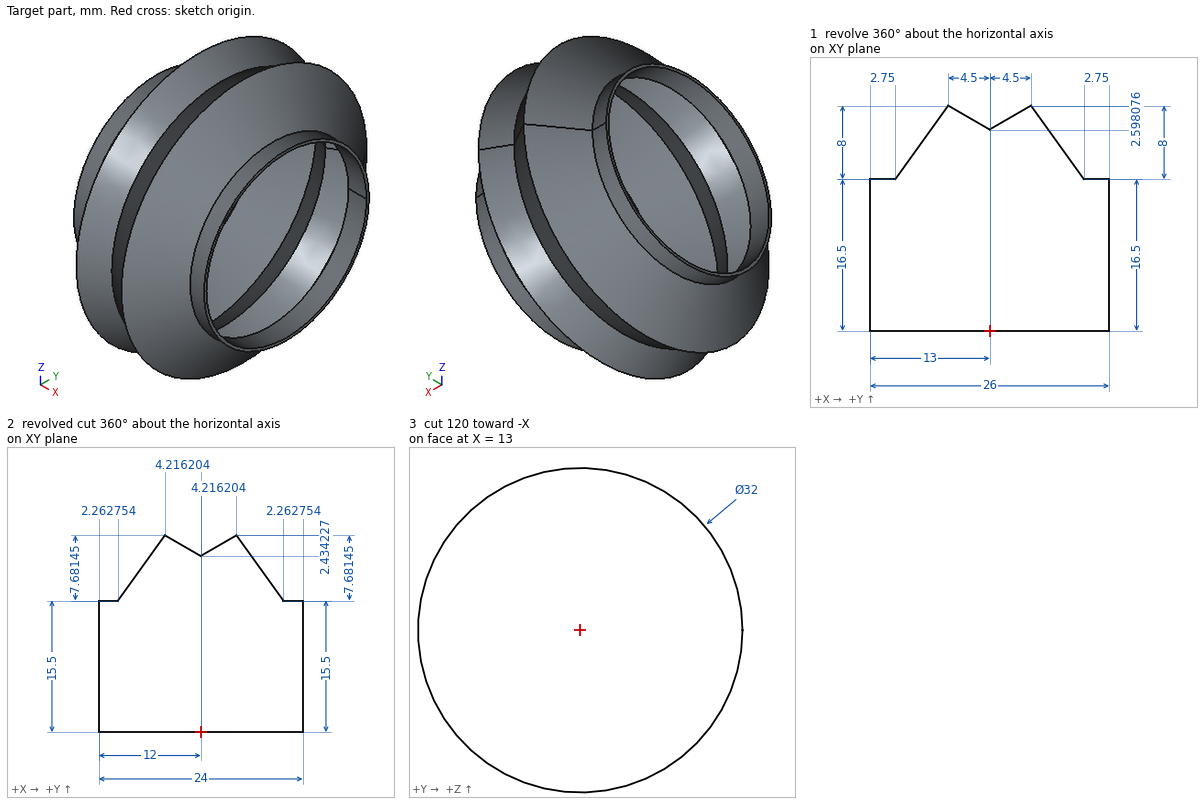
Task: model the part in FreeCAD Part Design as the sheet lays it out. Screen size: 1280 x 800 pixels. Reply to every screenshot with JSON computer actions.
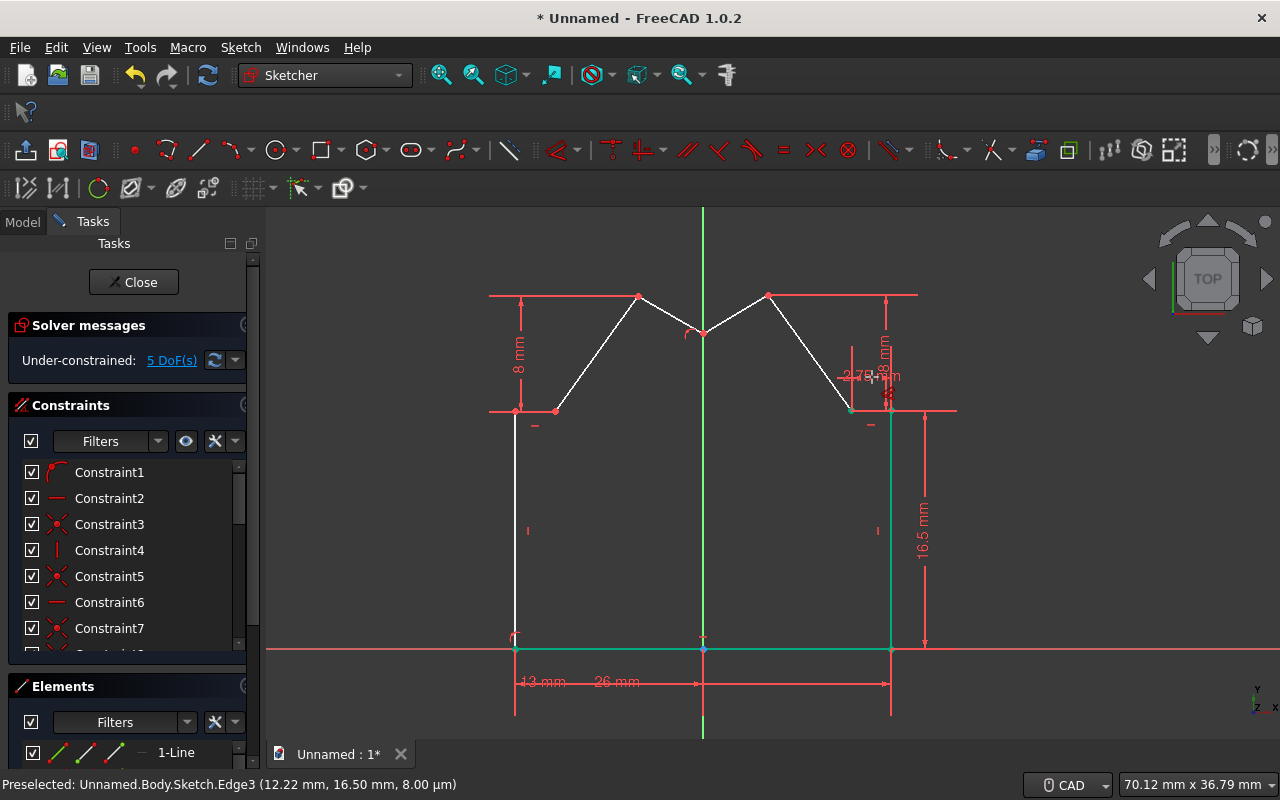
{"action": "left_click", "coordinate": [543, 412]}
{"action": "left_click", "coordinate": [535, 378]}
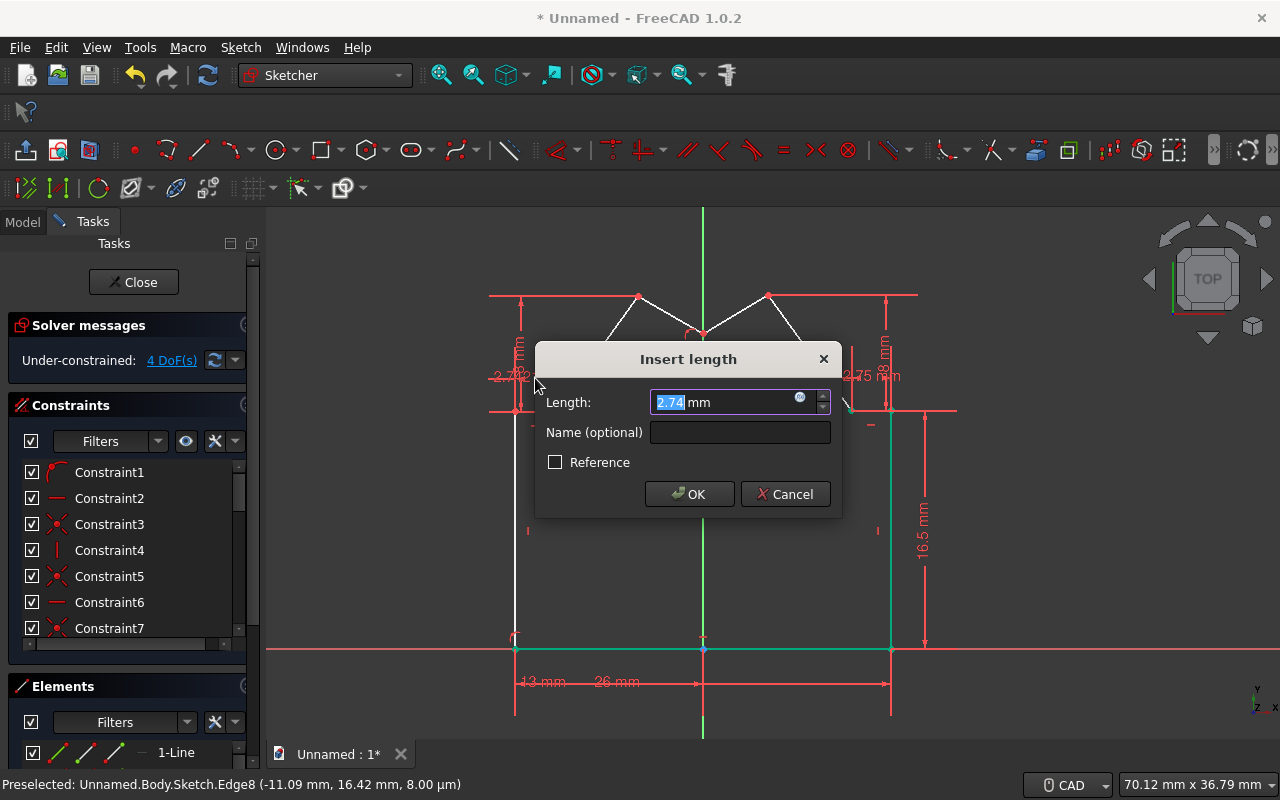
{"action": "type", "text": "2.75"}
{"action": "key", "text": "Return"}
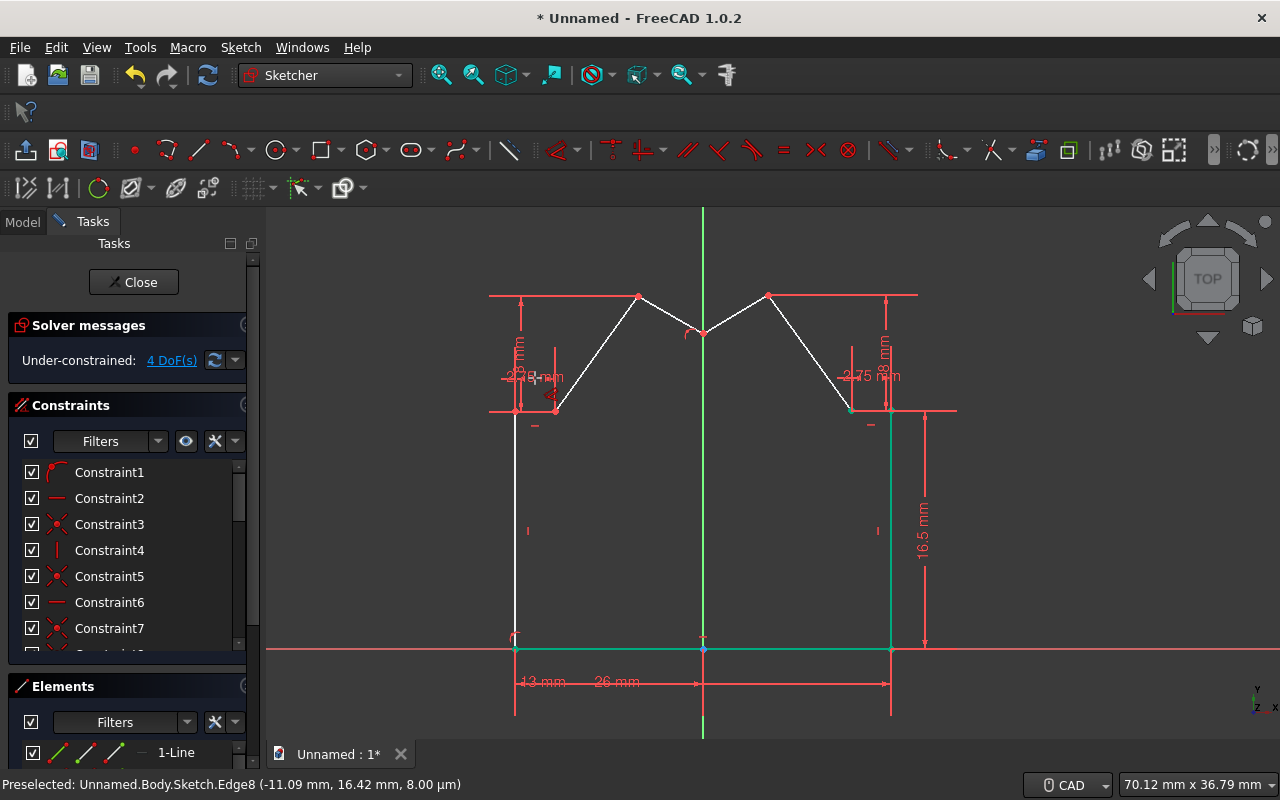
{"action": "left_click", "coordinate": [515, 483]}
{"action": "left_click", "coordinate": [481, 531]}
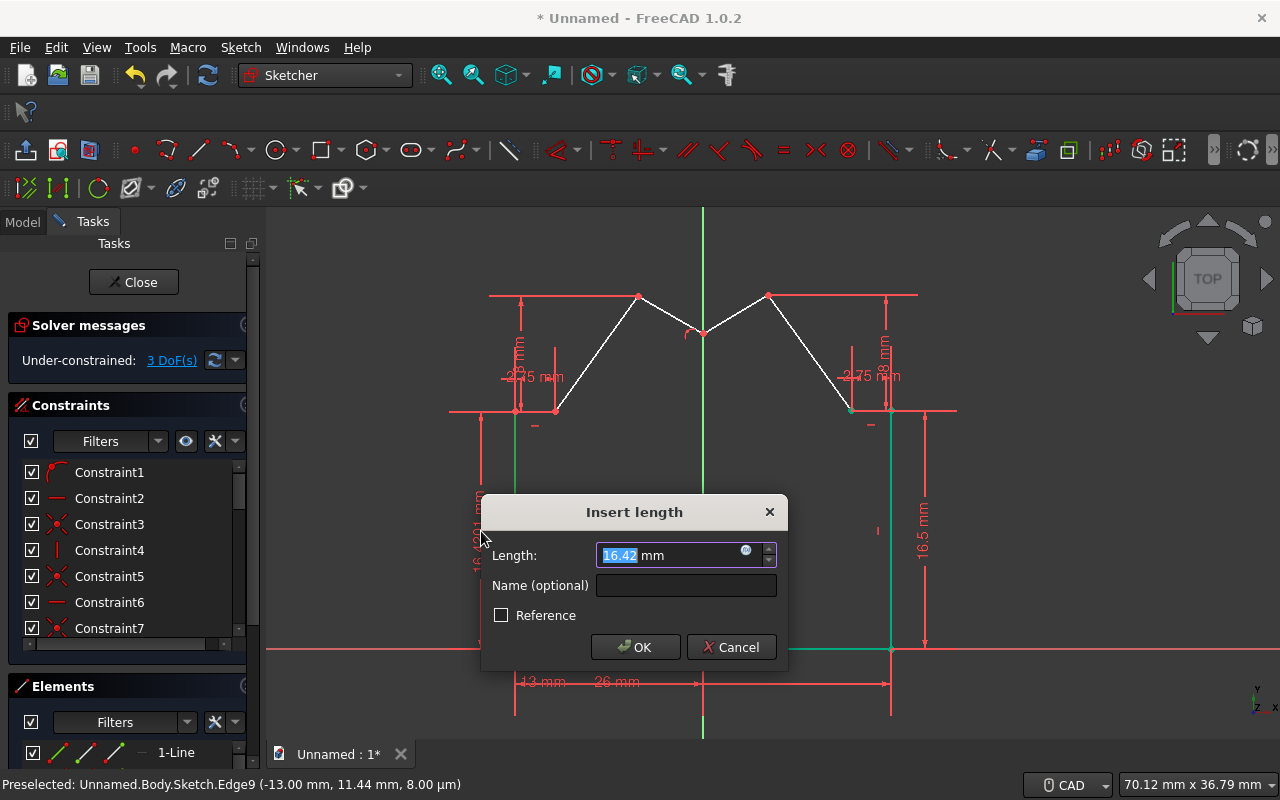
{"action": "type", "text": "16.5"}
{"action": "key", "text": "Return"}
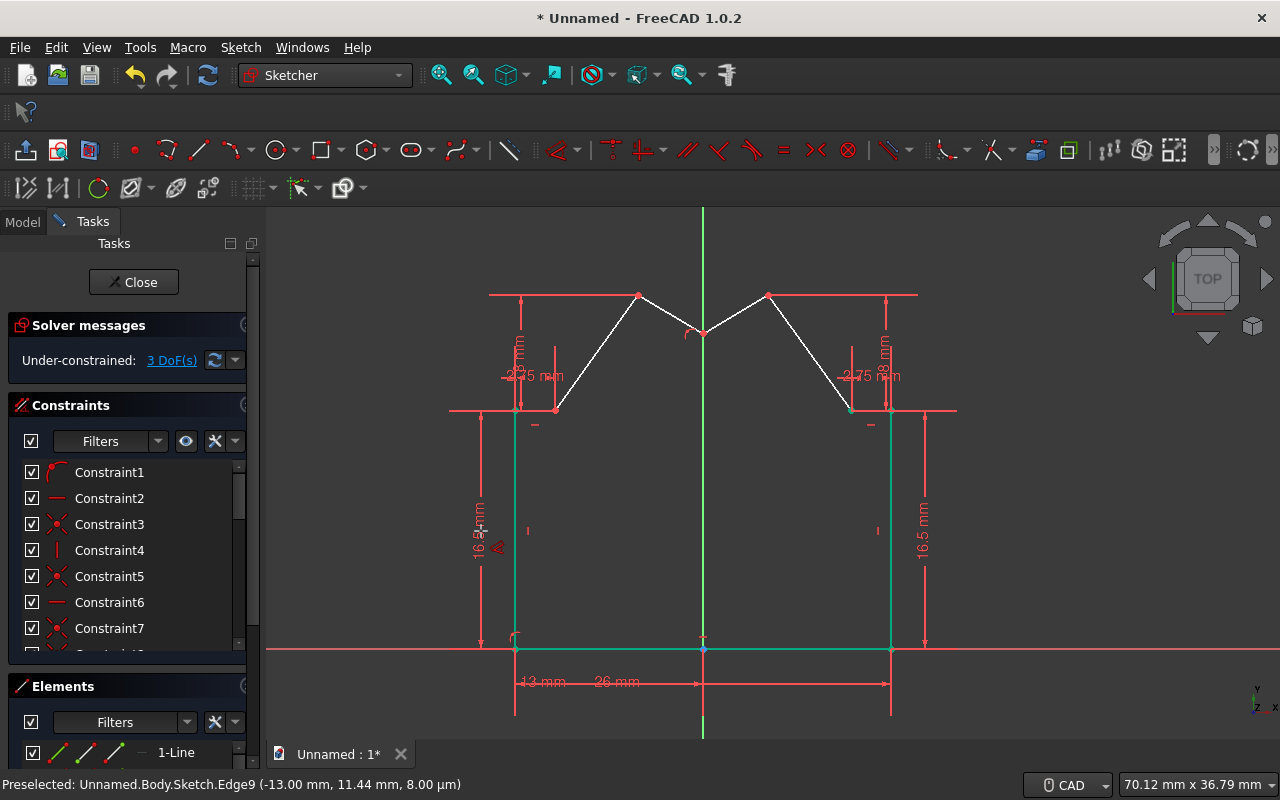
{"action": "left_click", "coordinate": [768, 295]}
{"action": "left_click", "coordinate": [736, 683]}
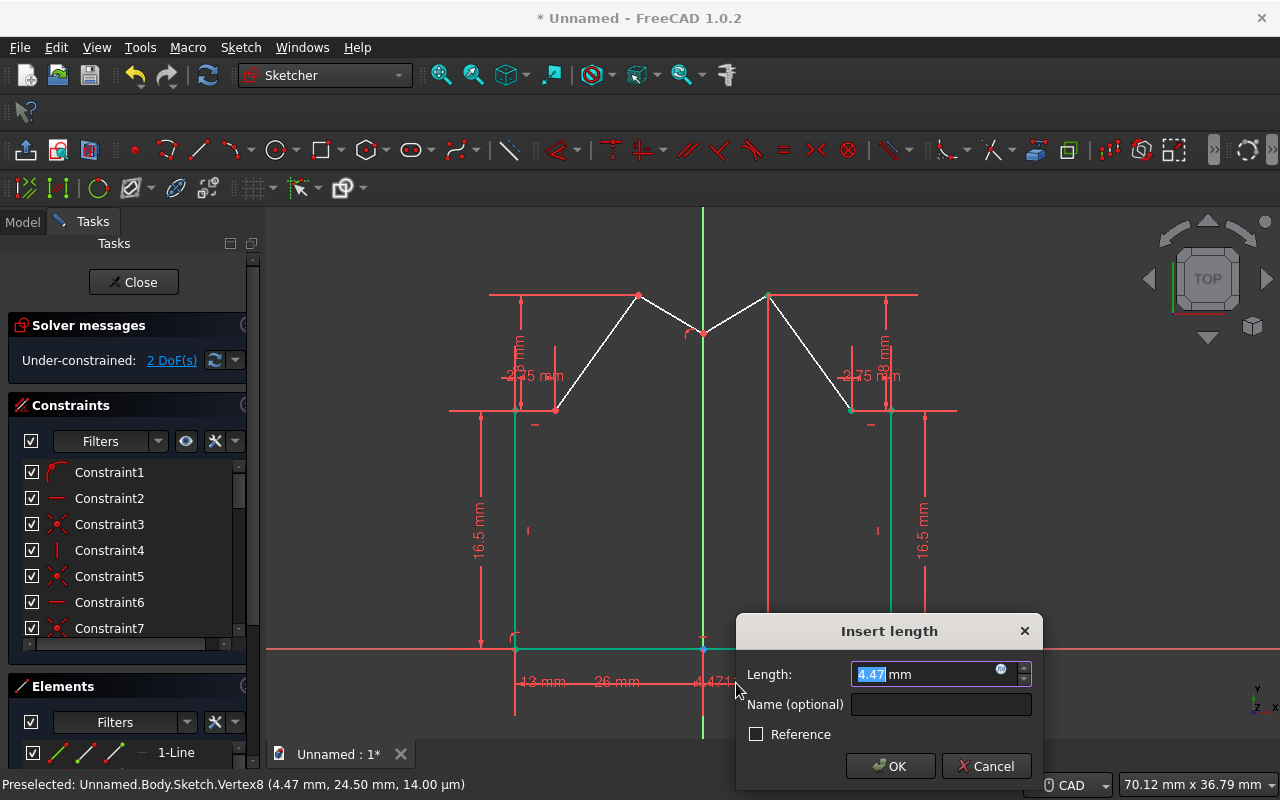
{"action": "type", "text": "4.5"}
{"action": "key", "text": "Return"}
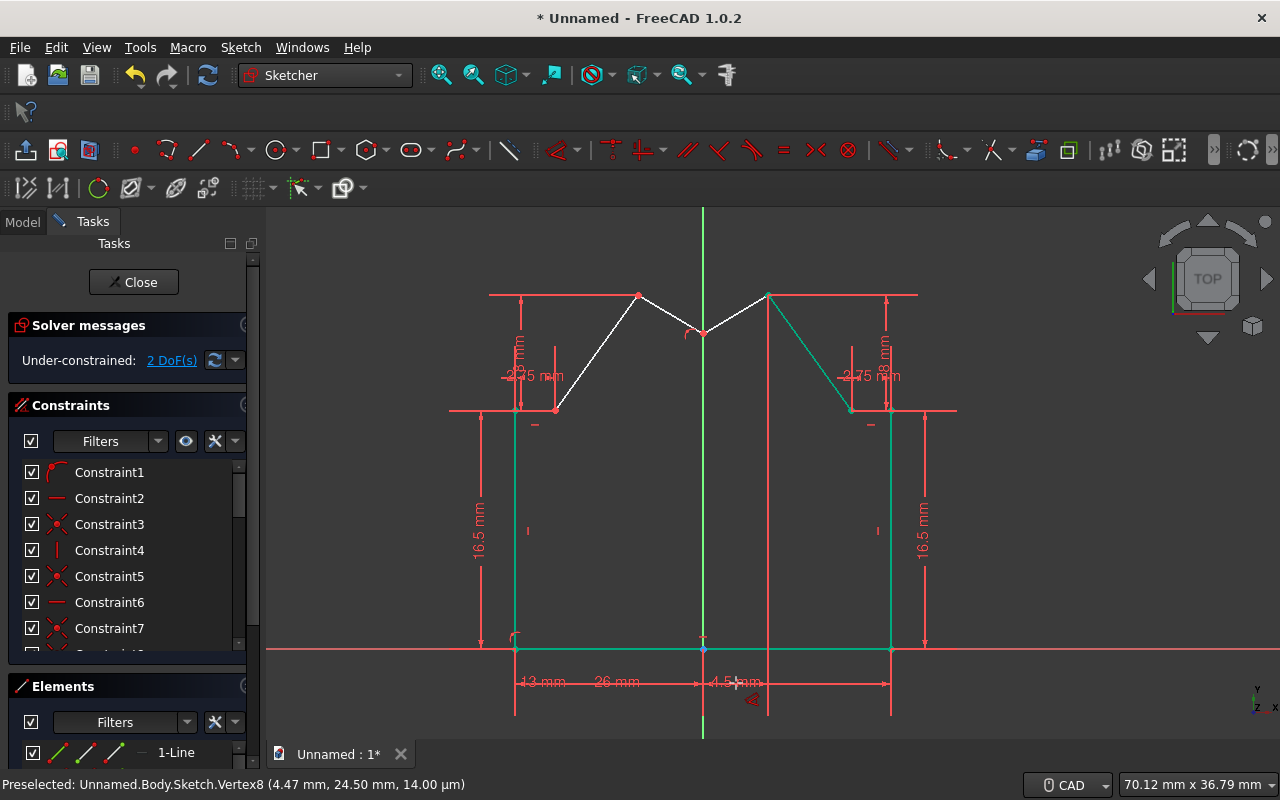
{"action": "left_click", "coordinate": [638, 295]}
{"action": "left_click", "coordinate": [671, 261]}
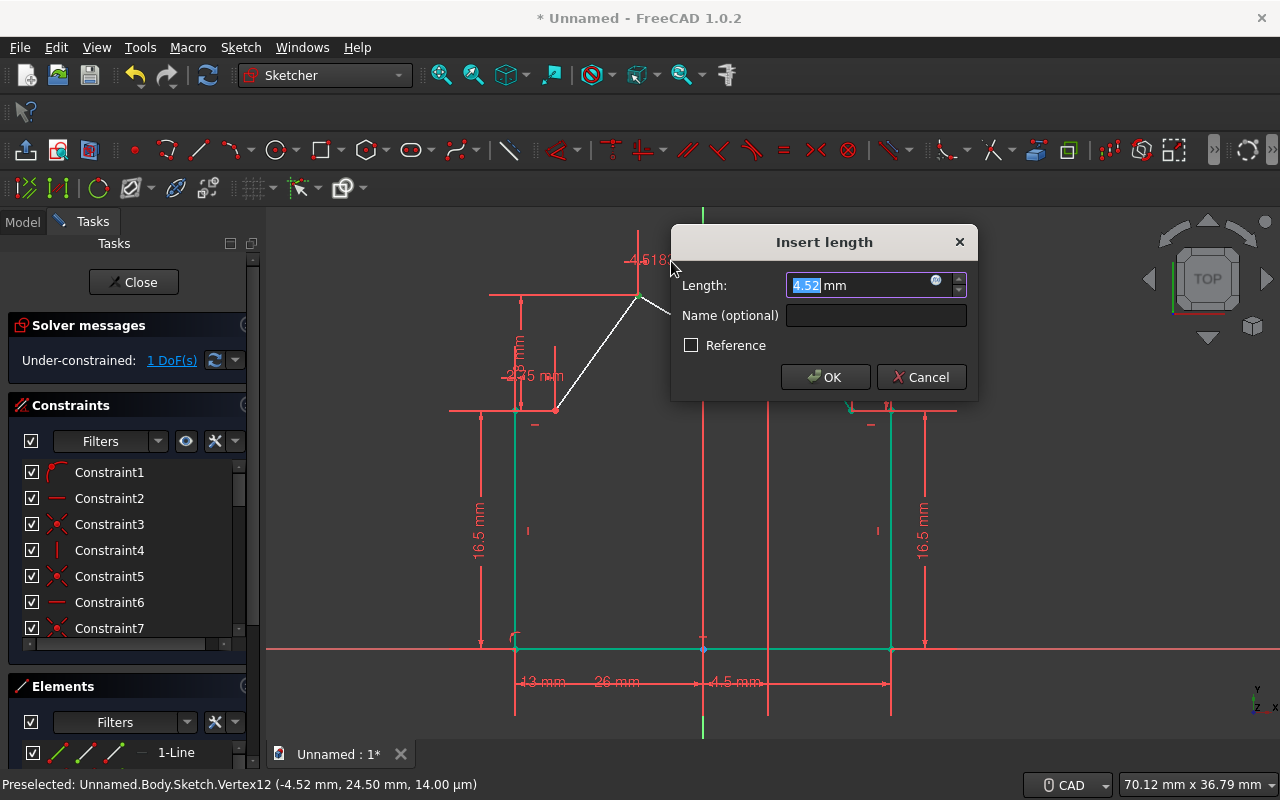
{"action": "type", "text": "4.5"}
{"action": "key", "text": "Return"}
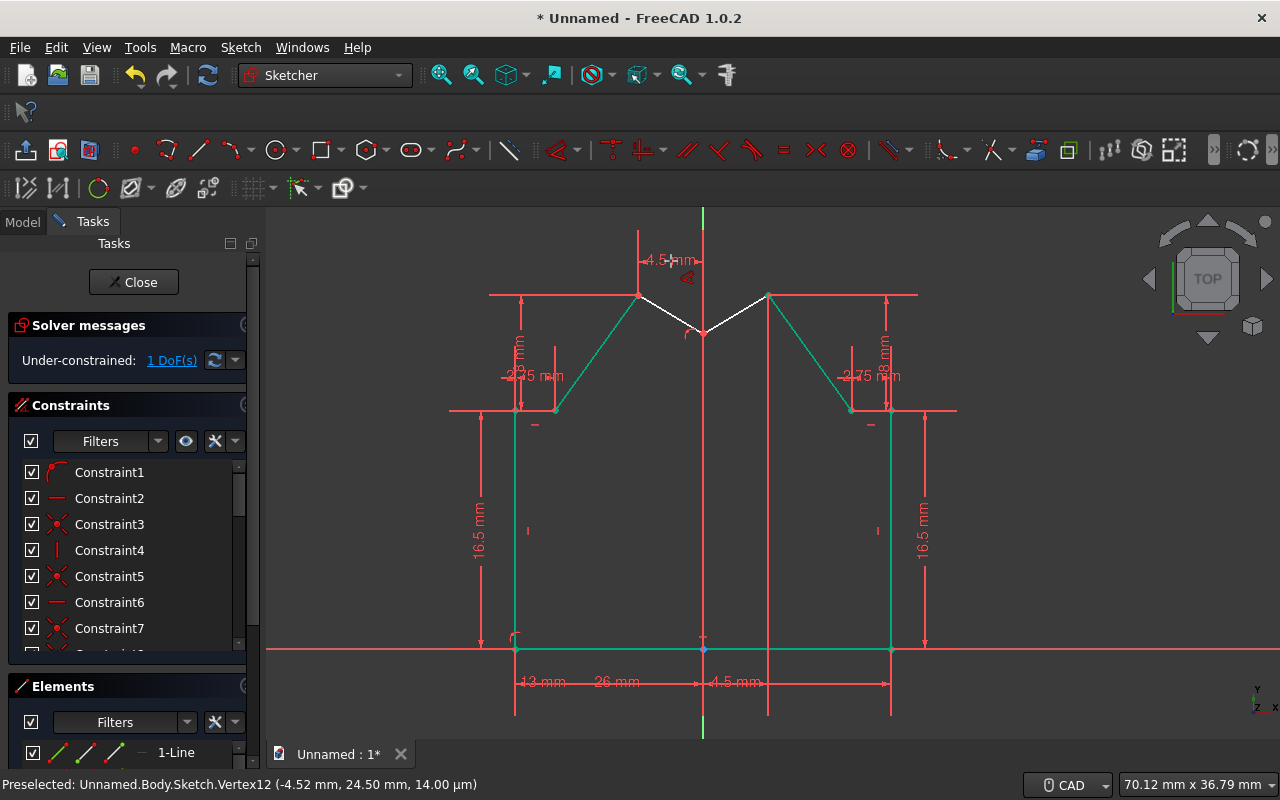
{"action": "left_click", "coordinate": [749, 307]}
{"action": "left_click", "coordinate": [802, 315]}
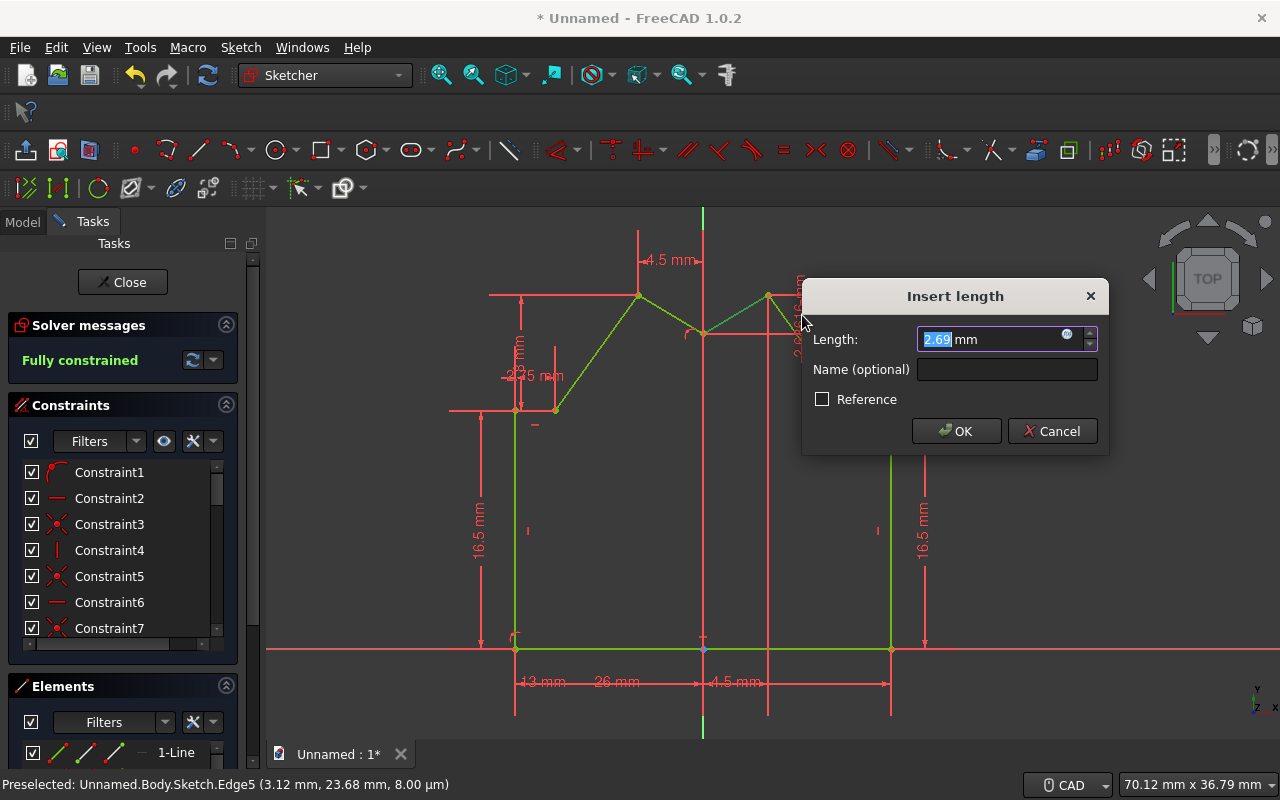
{"action": "type", "text": "2.598076"}
{"action": "key", "text": "Return"}
{"action": "key", "text": "Escape"}